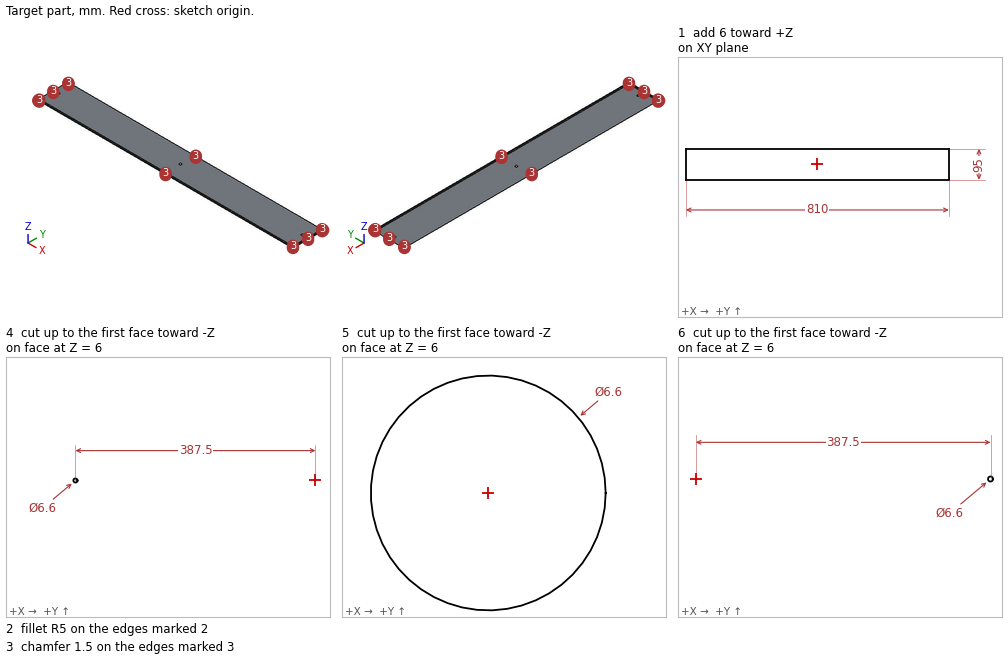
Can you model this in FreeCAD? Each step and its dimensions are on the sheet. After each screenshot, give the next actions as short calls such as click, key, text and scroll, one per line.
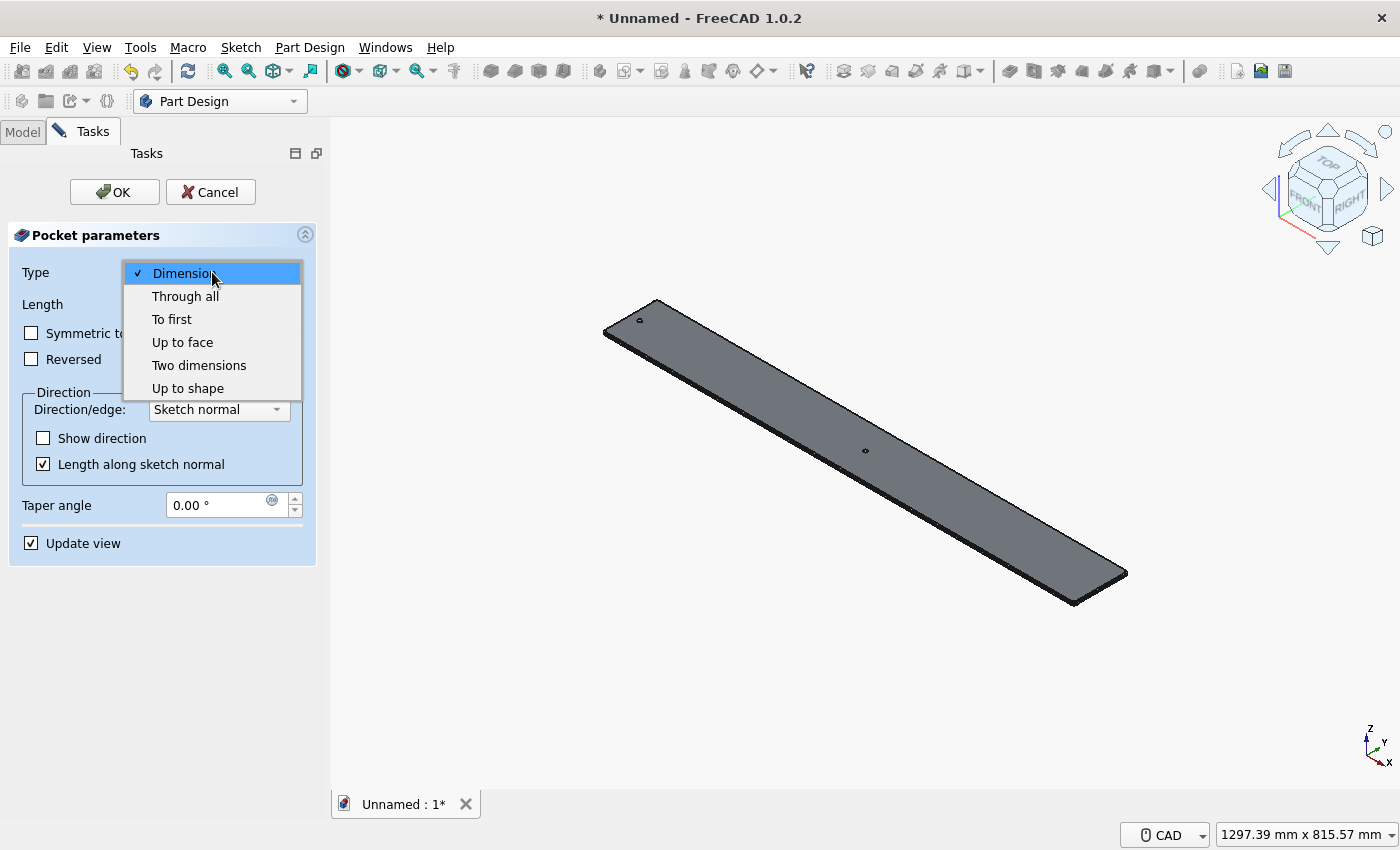
click(212, 320)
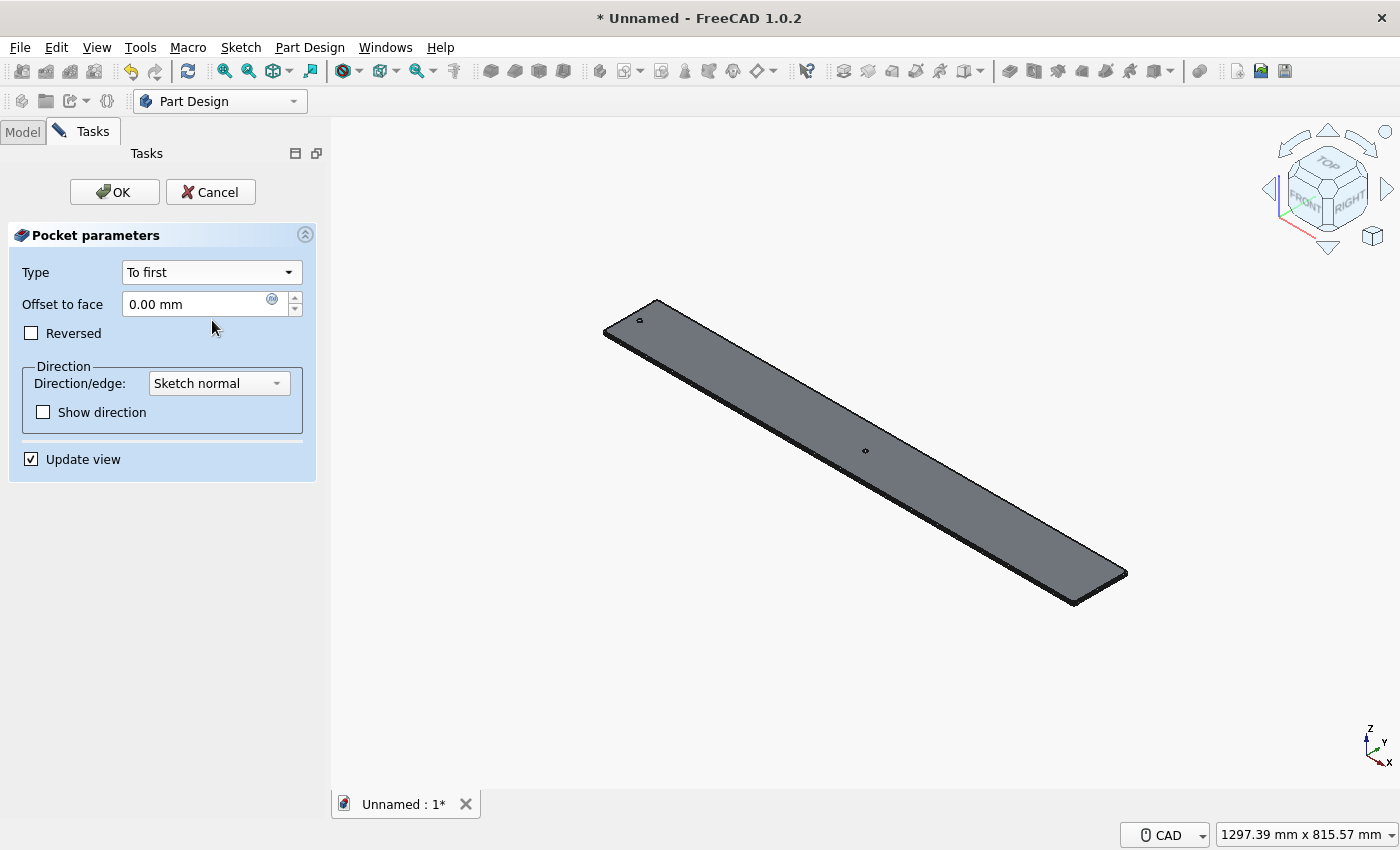
click(115, 192)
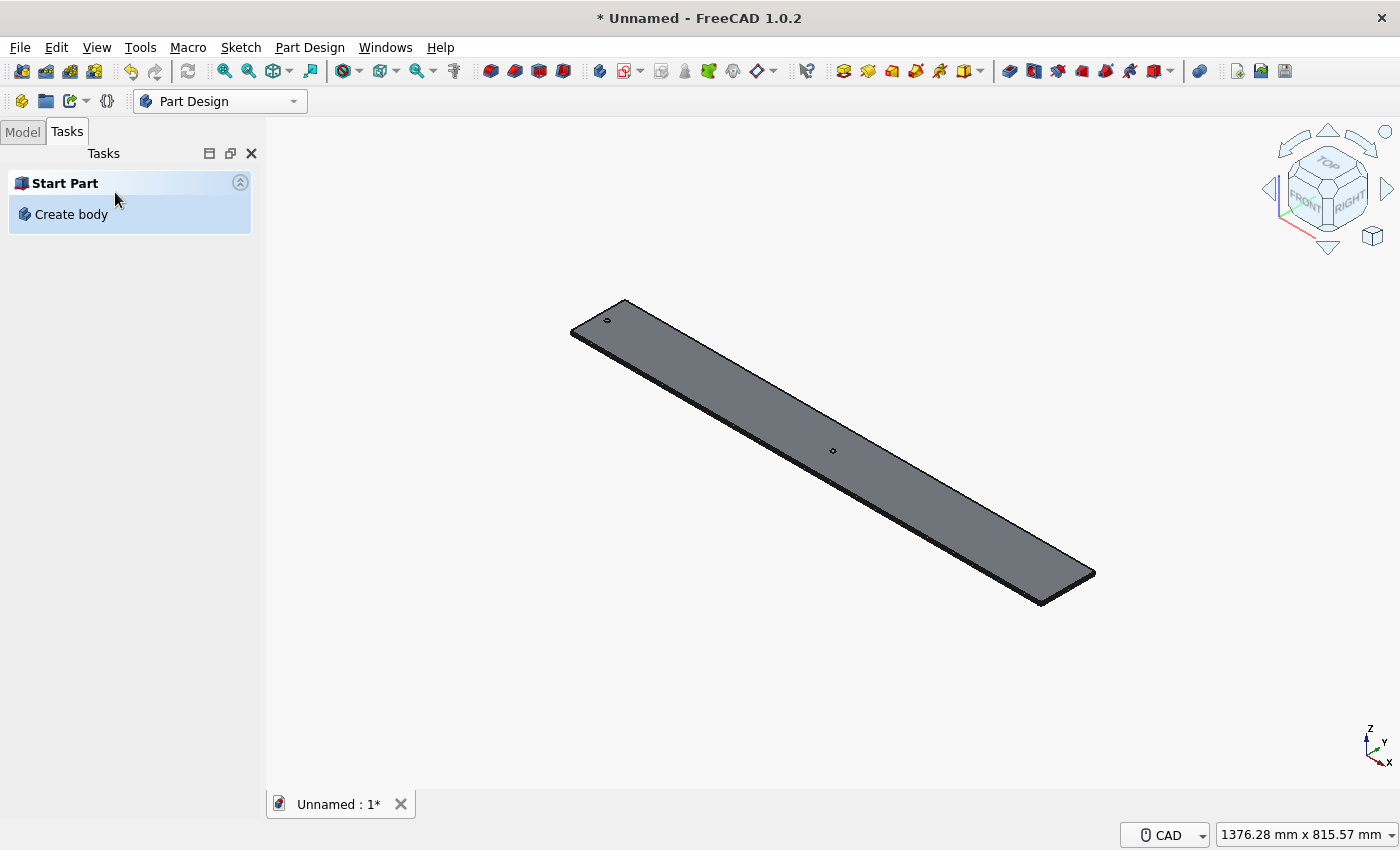
click(1035, 566)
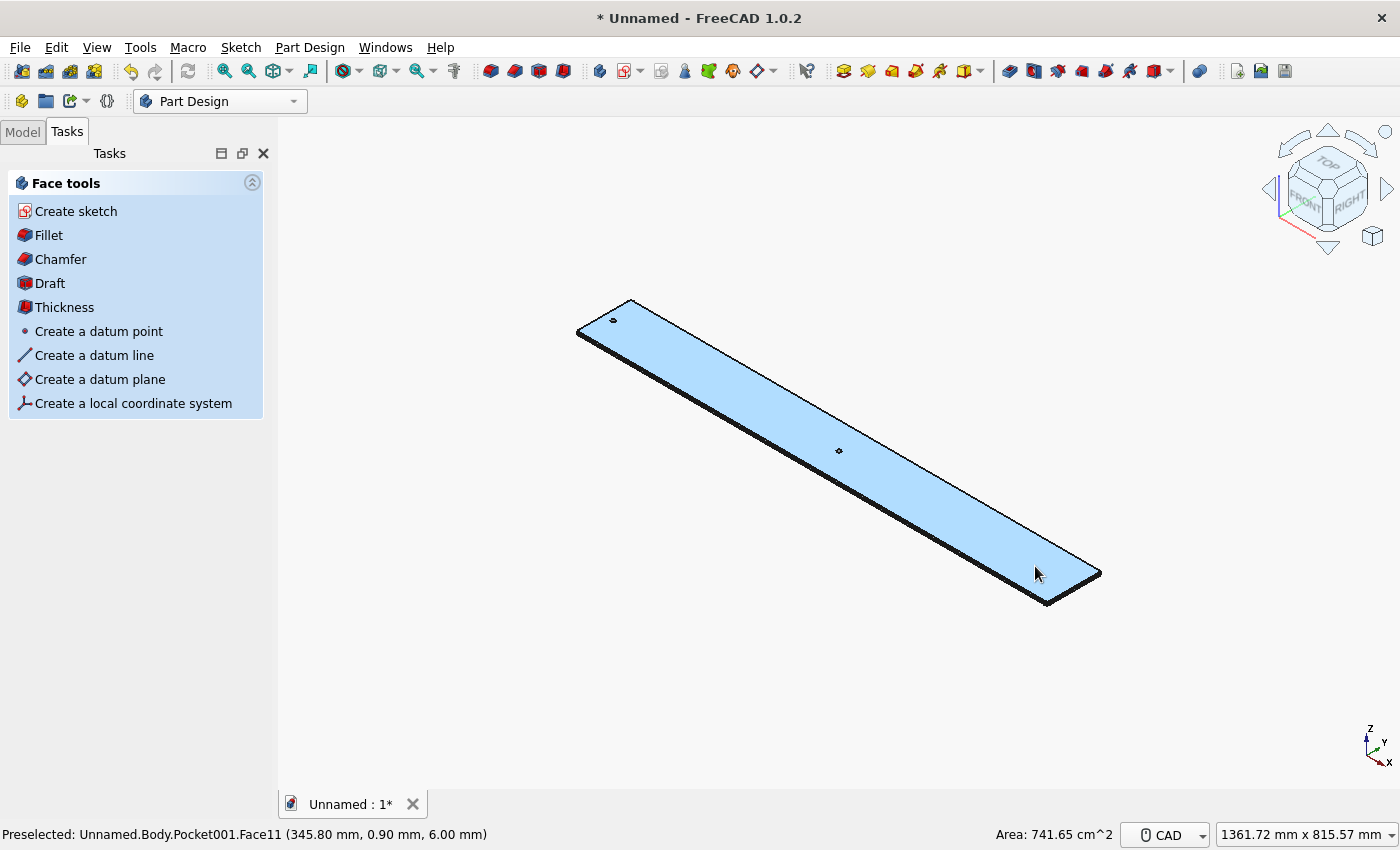
click(624, 72)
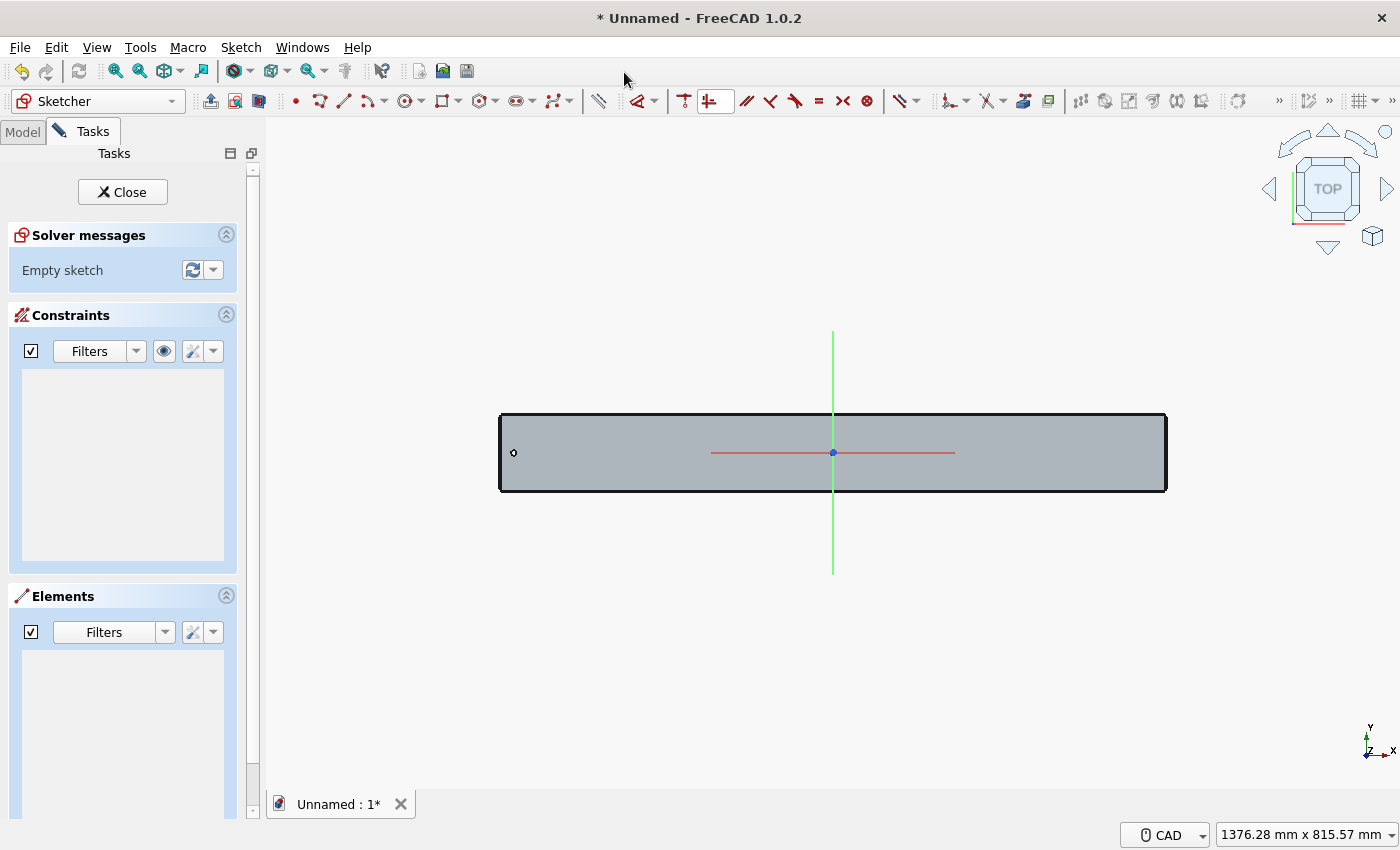
scroll(1173, 453, up, 15)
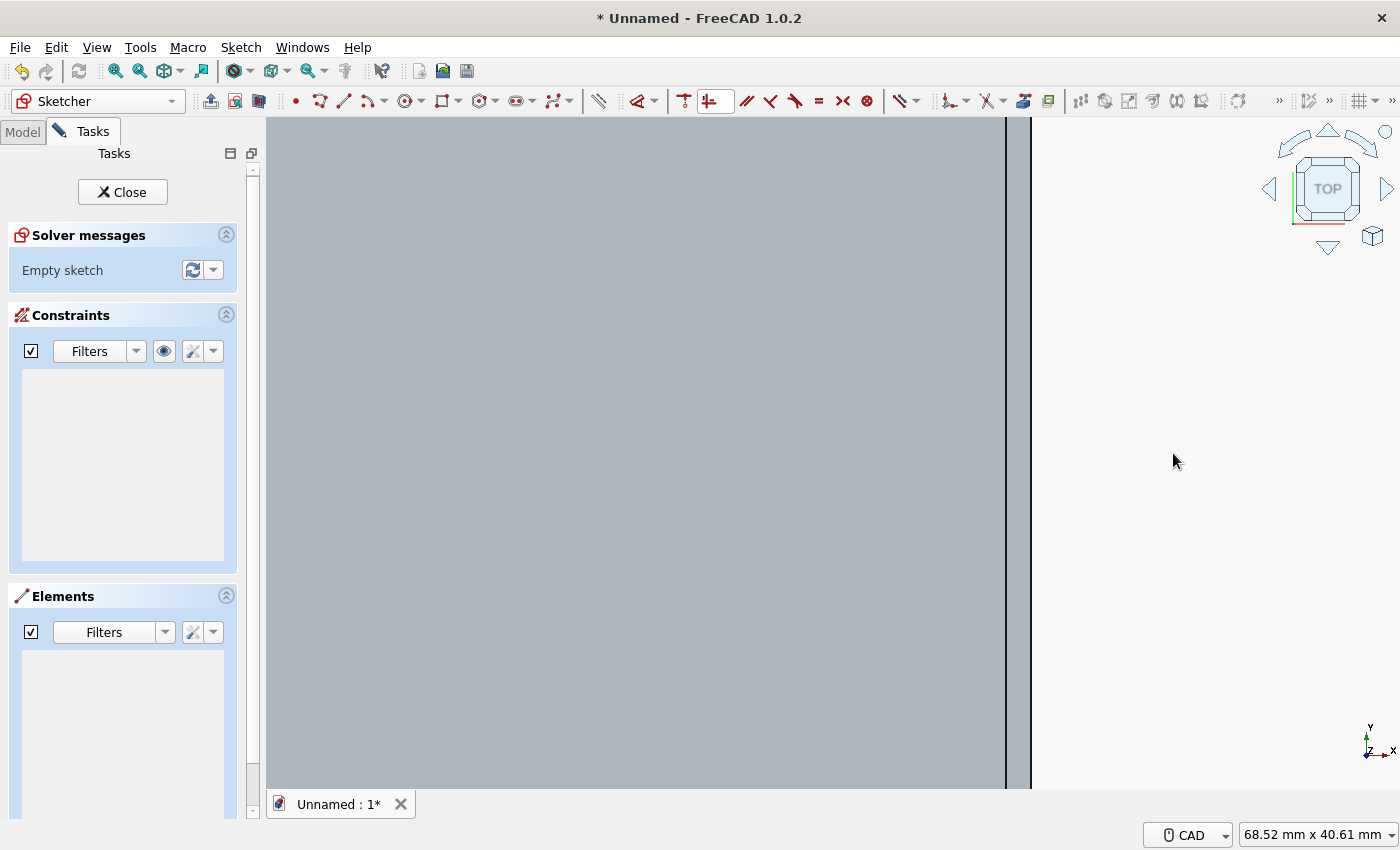
scroll(734, 440, up, 7)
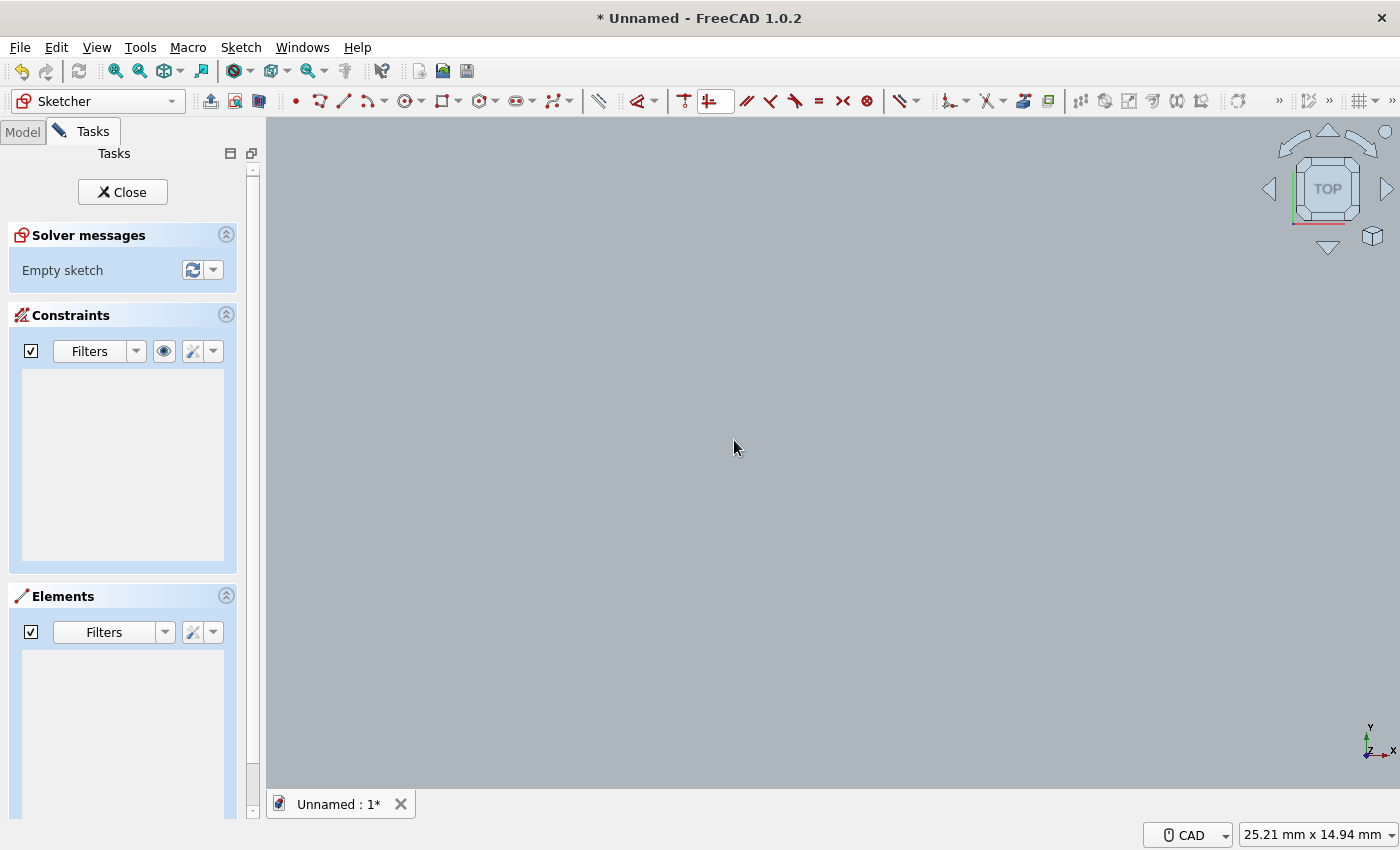
key(g)
key(c)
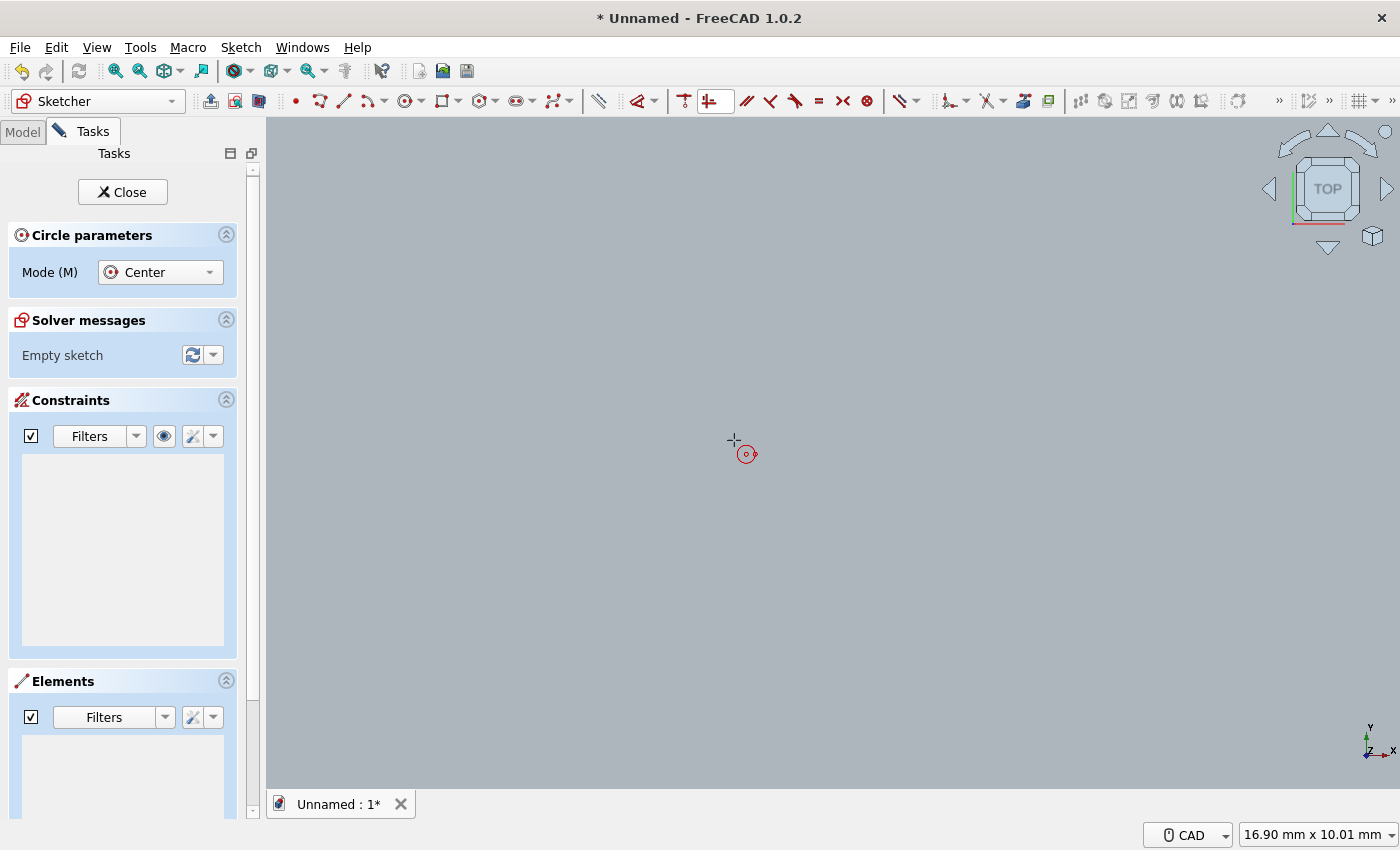
click(764, 452)
move(920, 296)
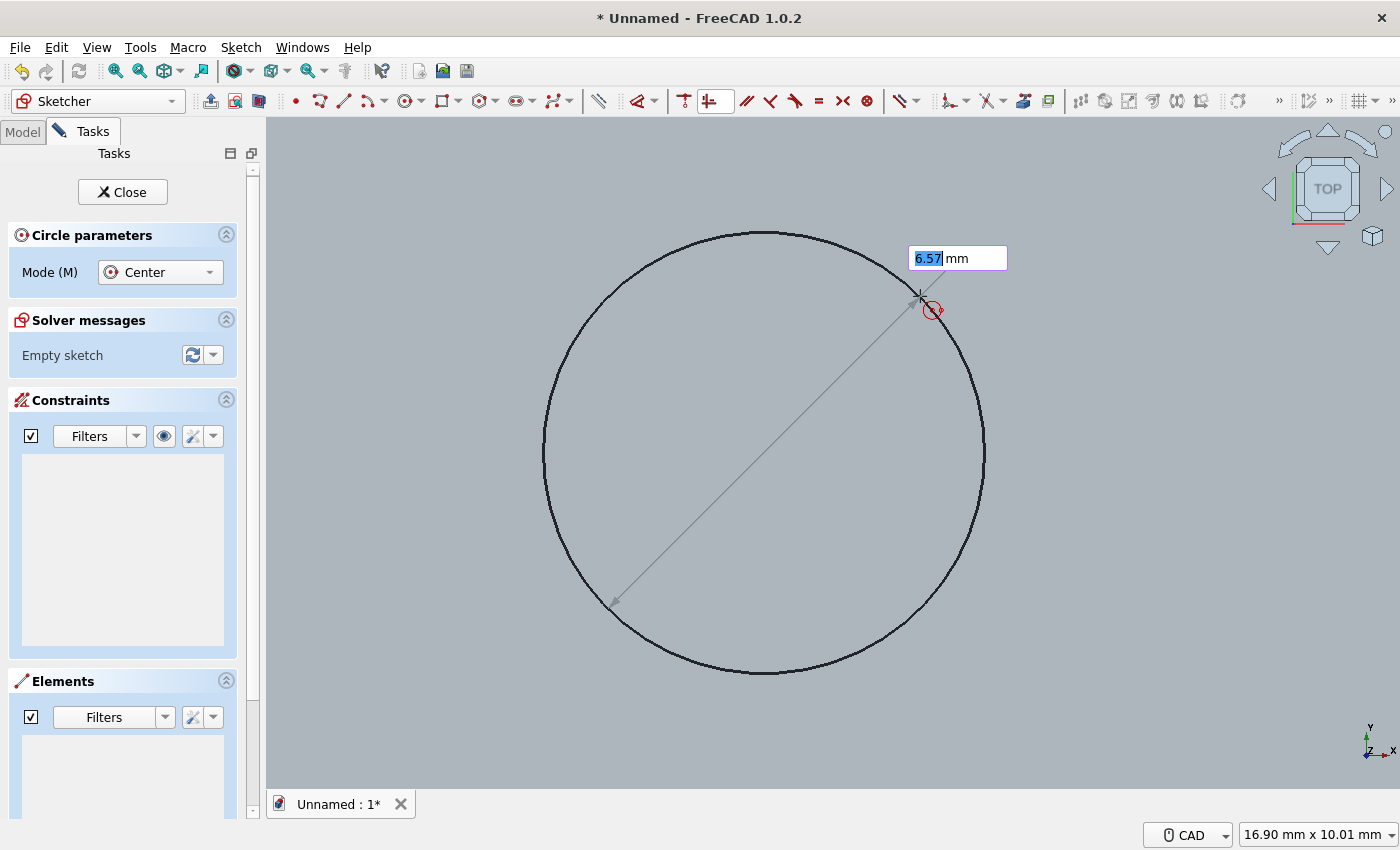
text(6.6)
key(Return)
key(Escape)